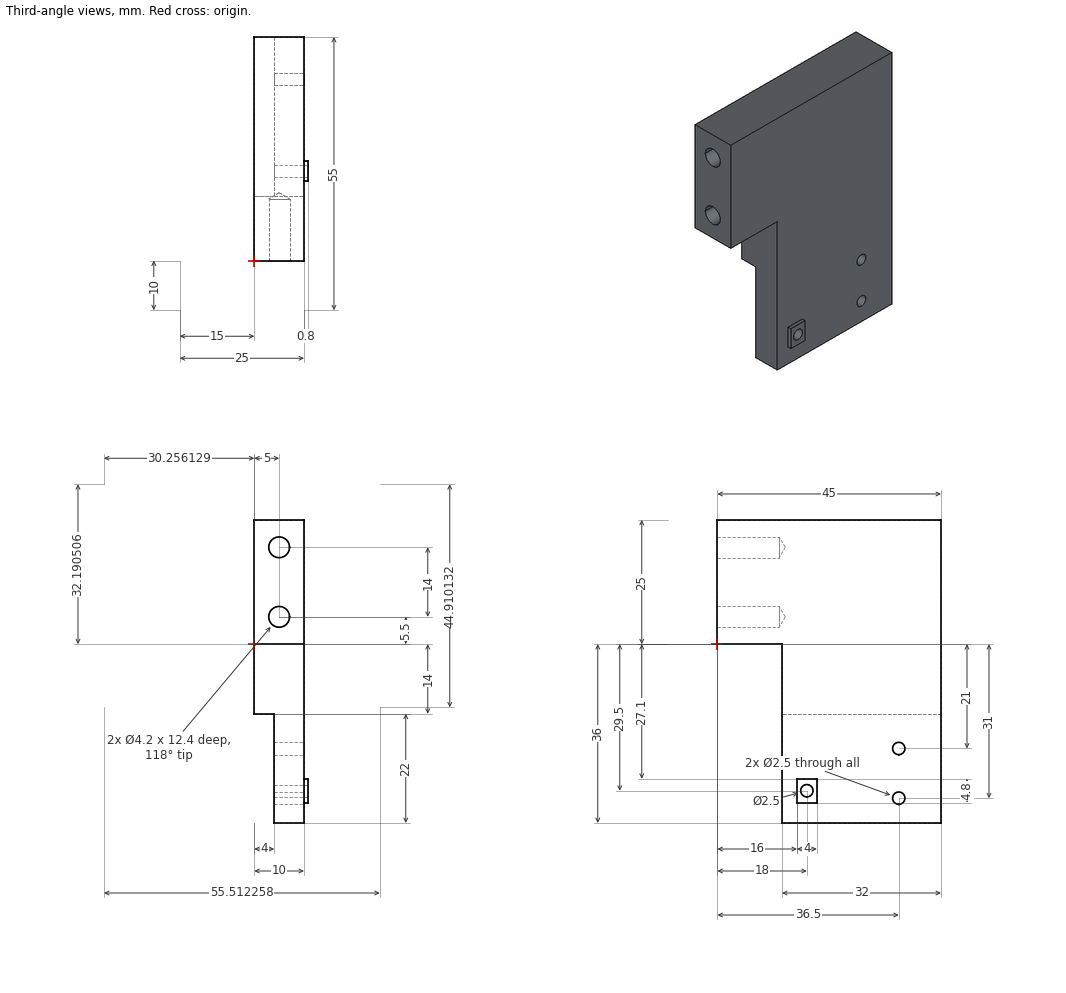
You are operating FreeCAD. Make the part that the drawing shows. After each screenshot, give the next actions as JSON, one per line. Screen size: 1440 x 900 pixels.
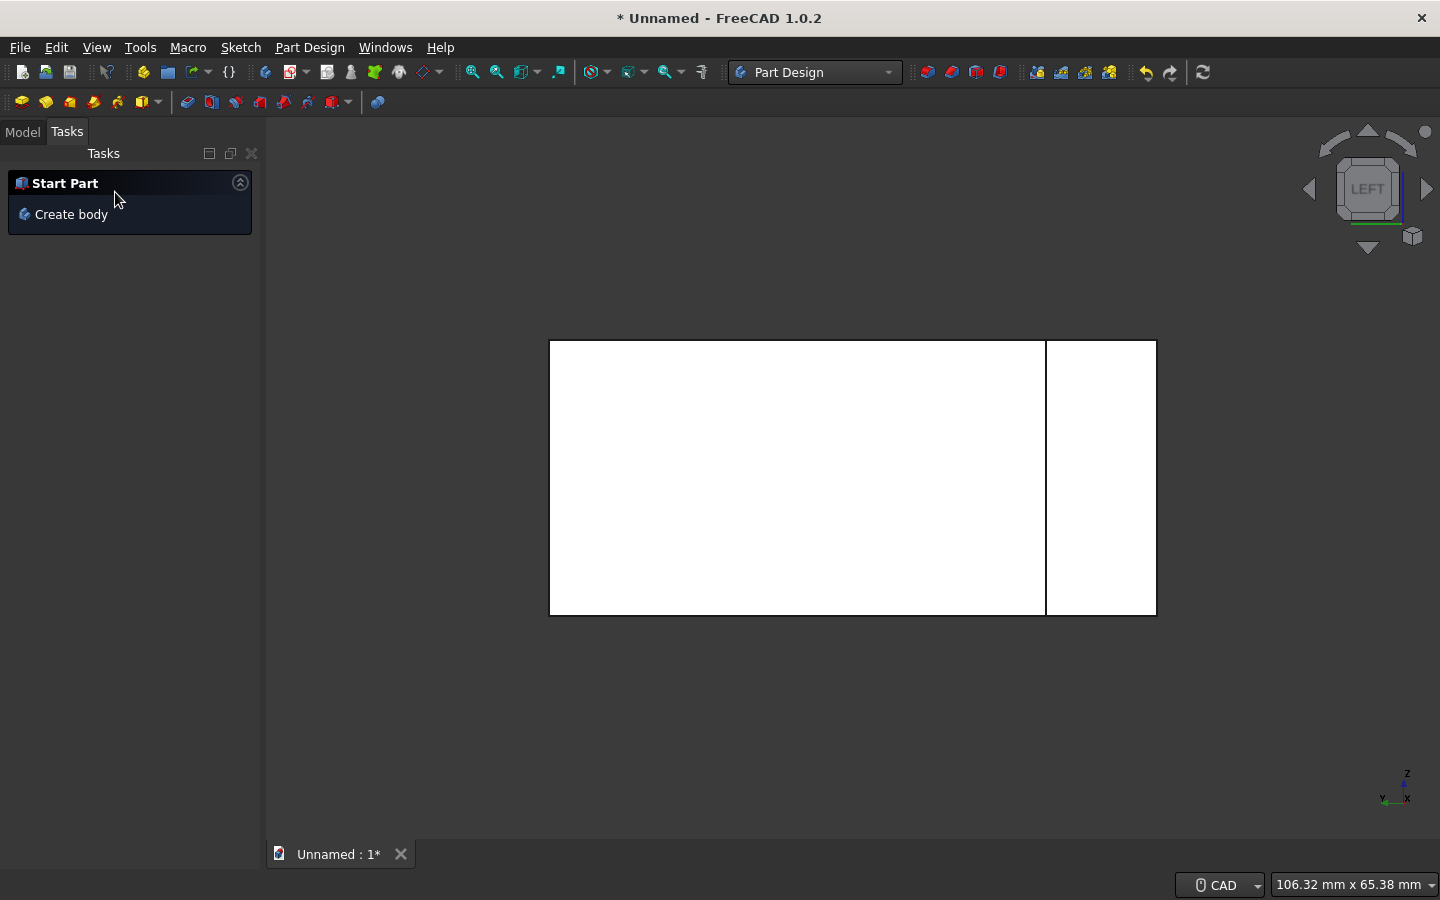
{"action": "left_click", "coordinate": [727, 477]}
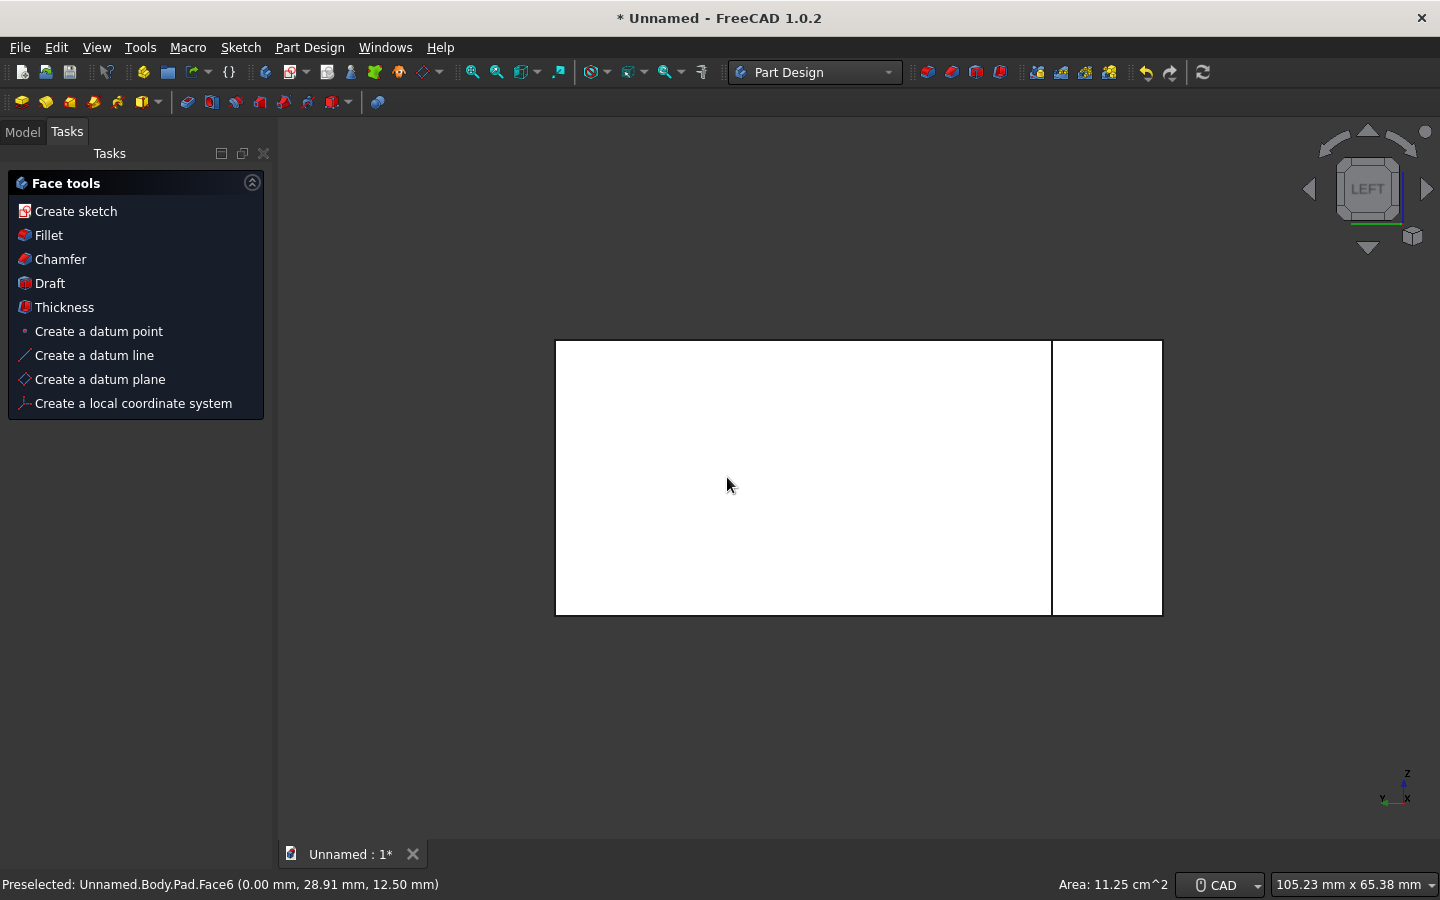
{"action": "left_click", "coordinate": [290, 72]}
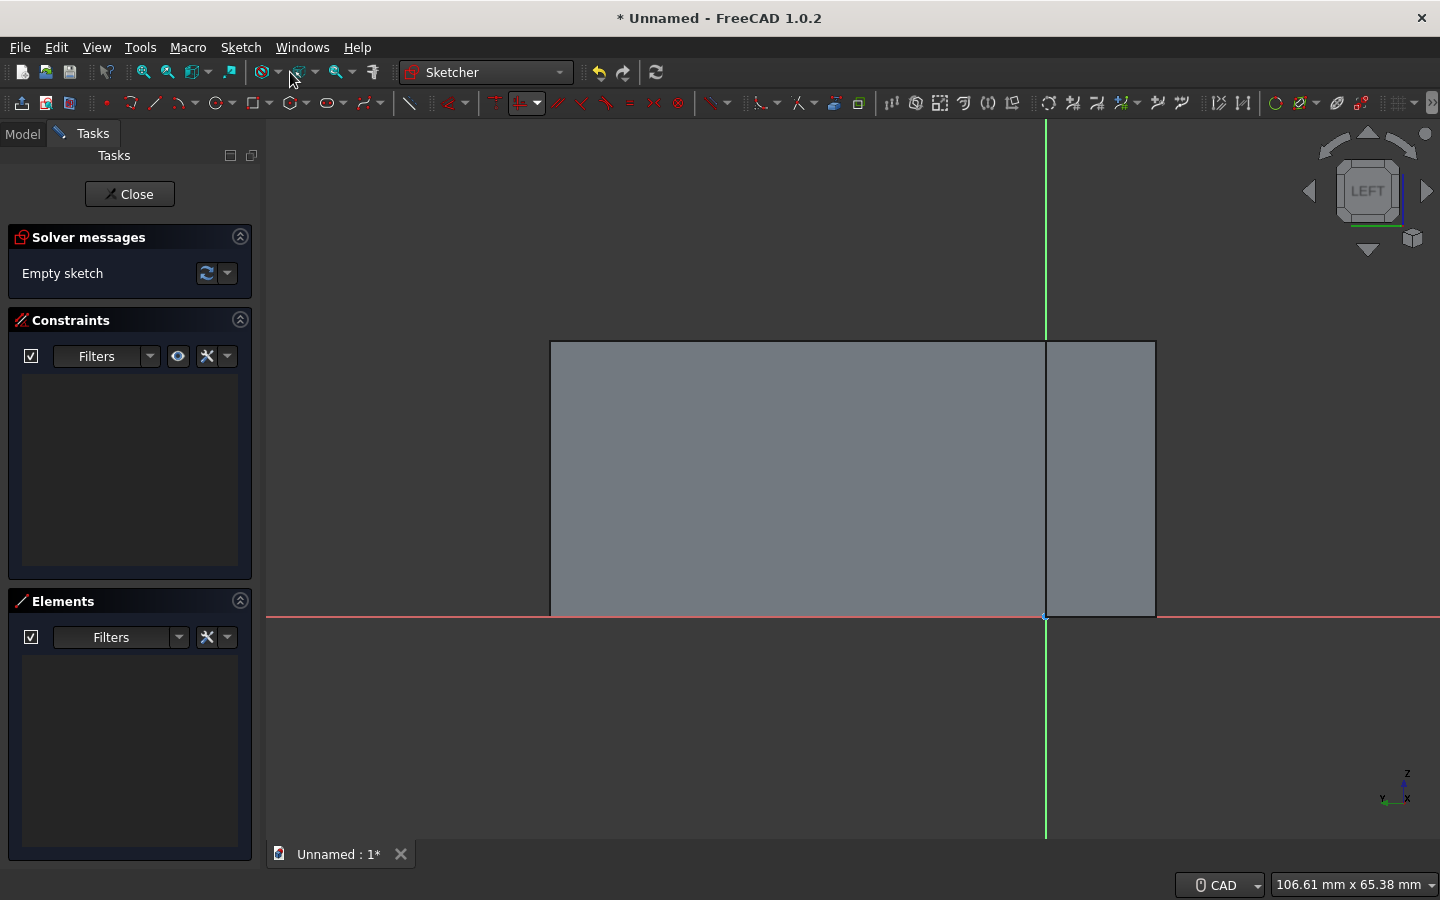
{"action": "key", "text": "q s"}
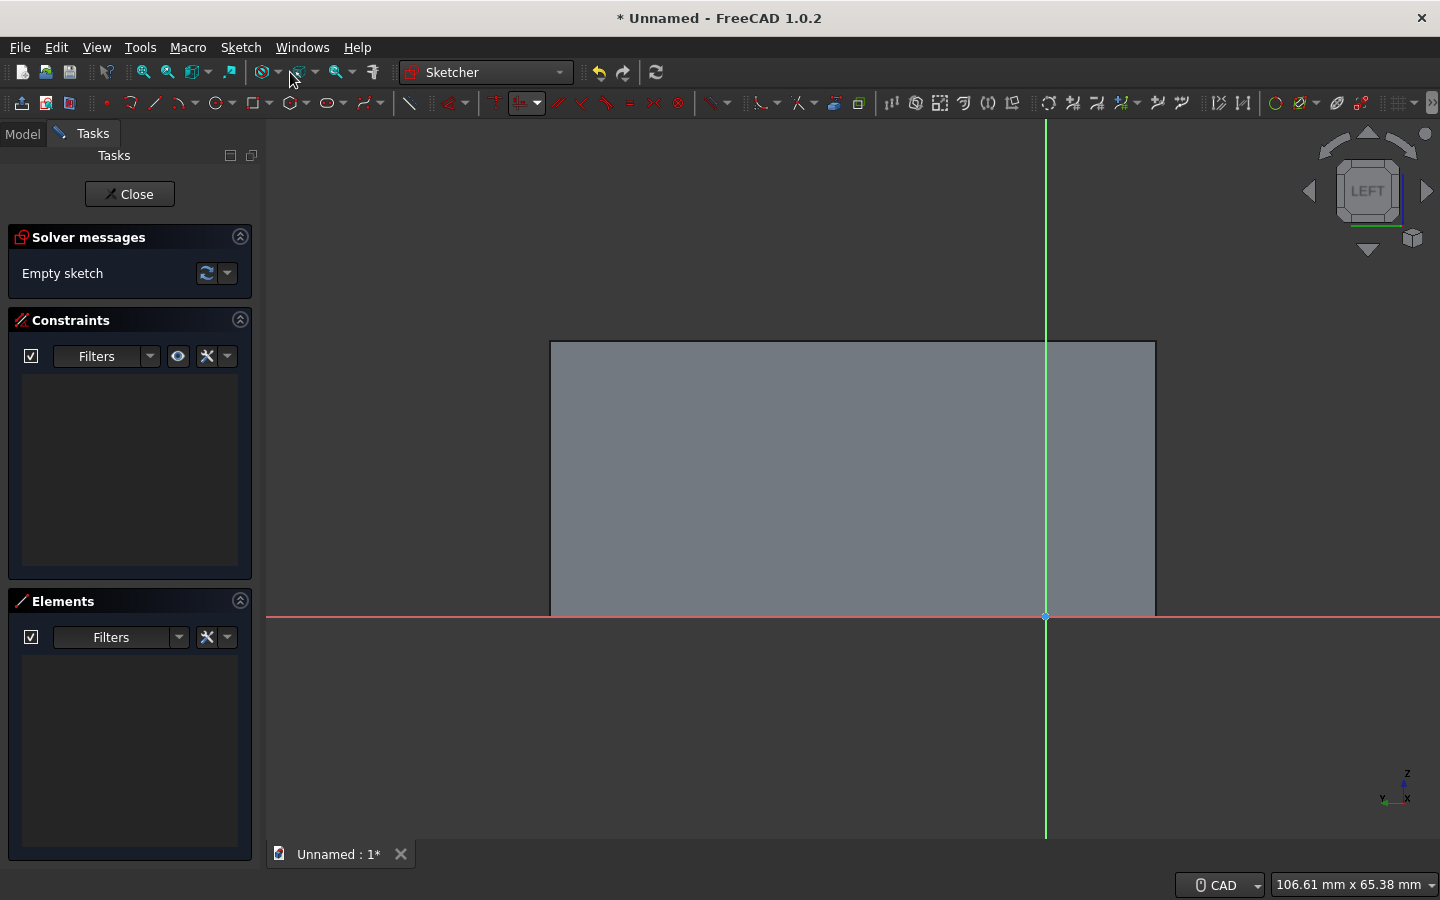
{"action": "scroll", "coordinate": [757, 147], "scroll_direction": "down", "scroll_amount": 2}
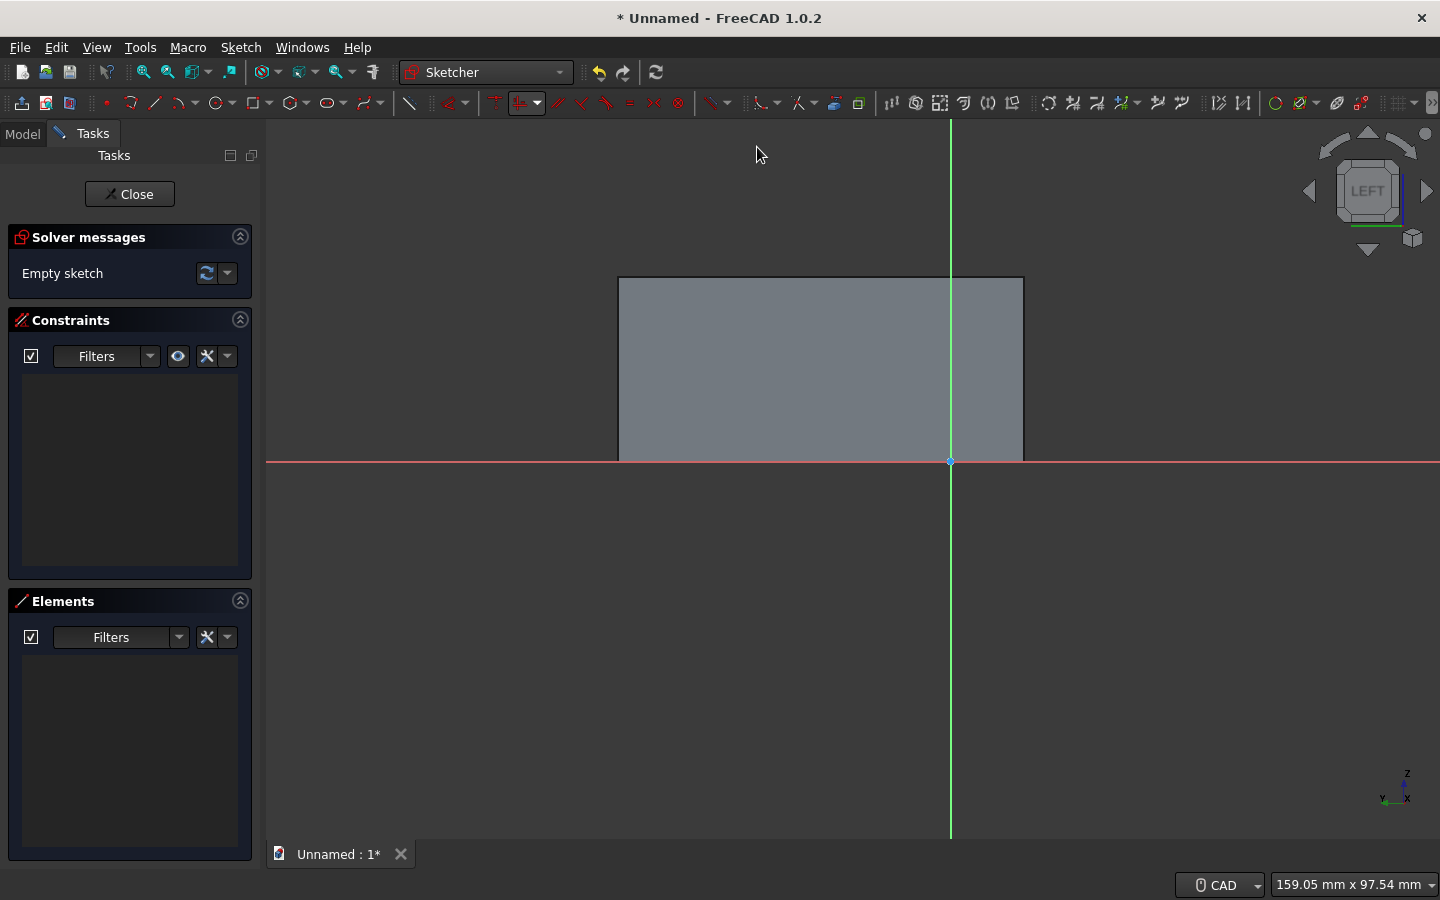
{"action": "scroll", "coordinate": [785, 735], "scroll_direction": "up", "scroll_amount": 3}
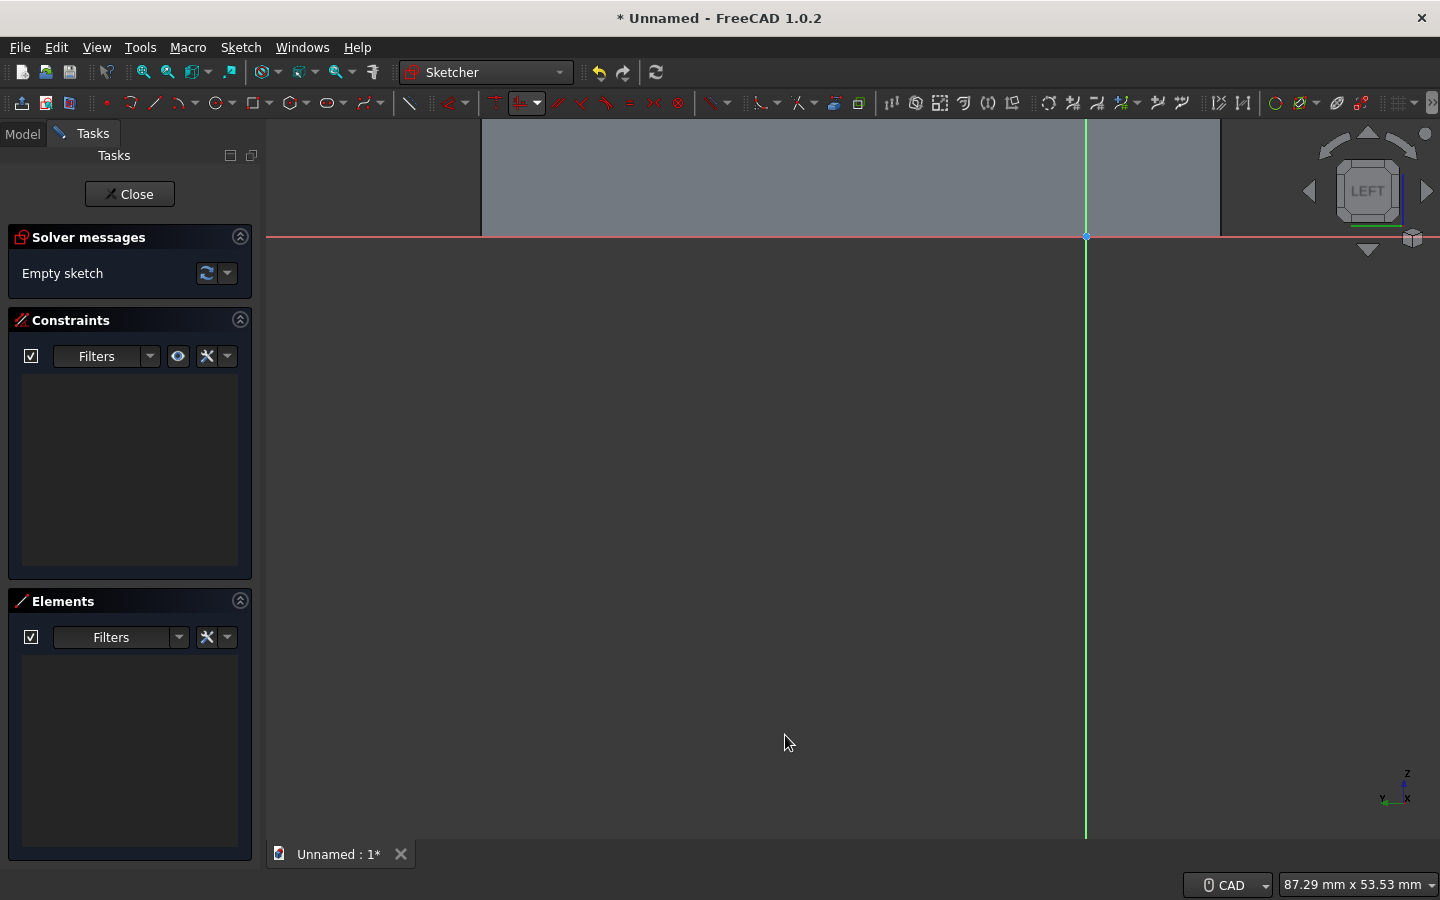
{"action": "left_click", "coordinate": [254, 104]}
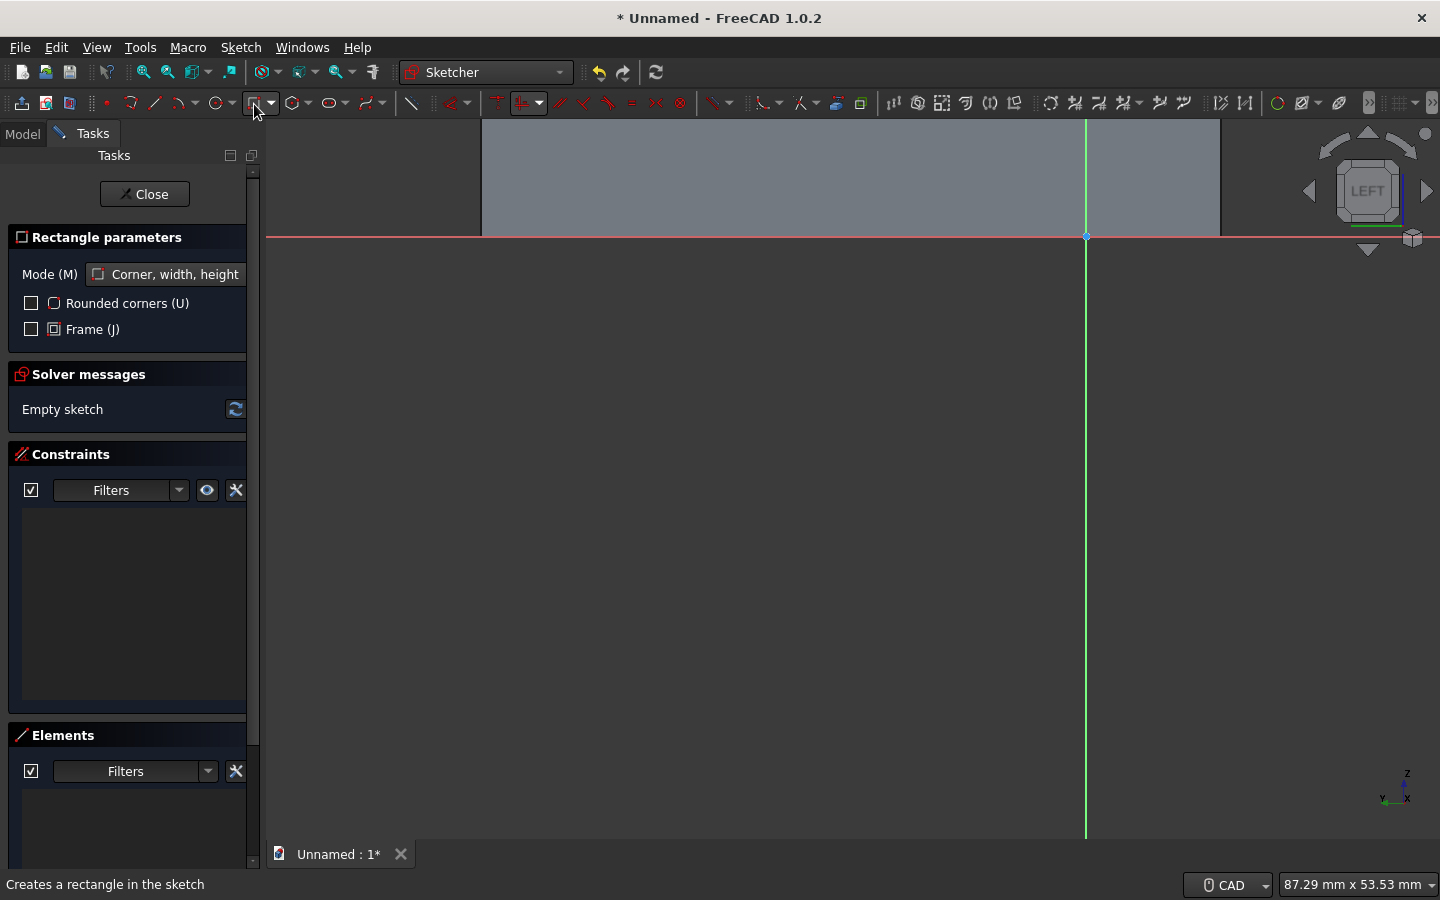
{"action": "left_click", "coordinate": [481, 237]}
{"action": "mouse_move", "coordinate": [912, 721]}